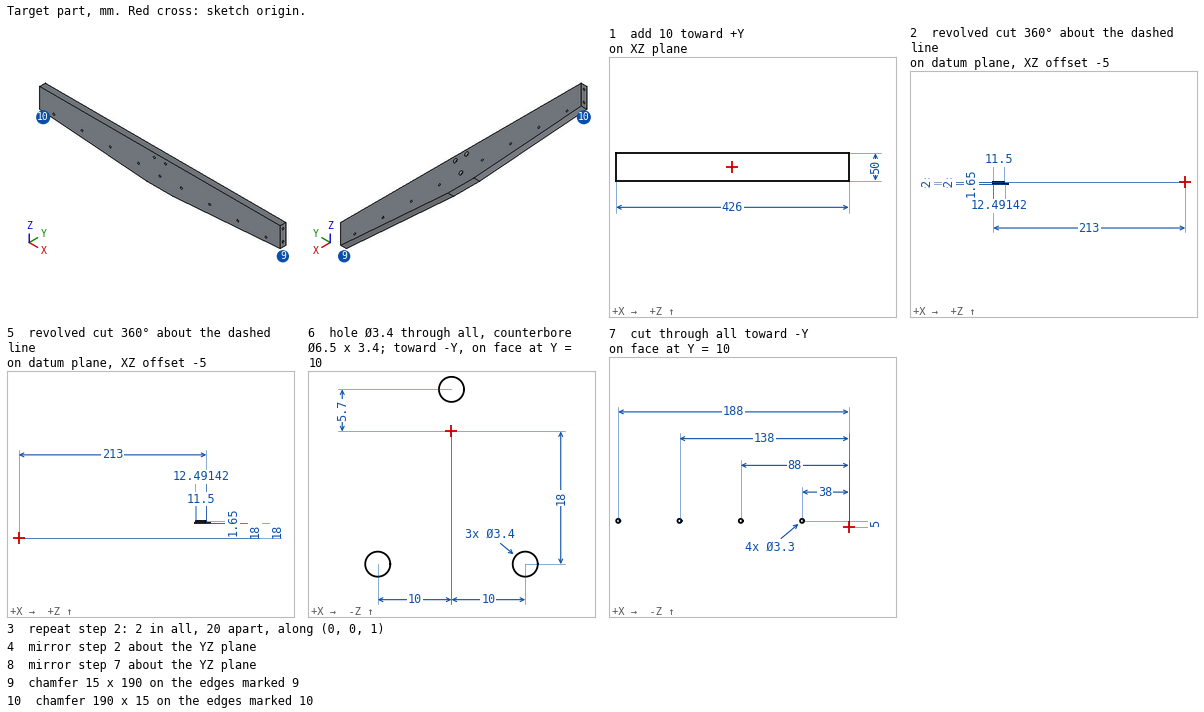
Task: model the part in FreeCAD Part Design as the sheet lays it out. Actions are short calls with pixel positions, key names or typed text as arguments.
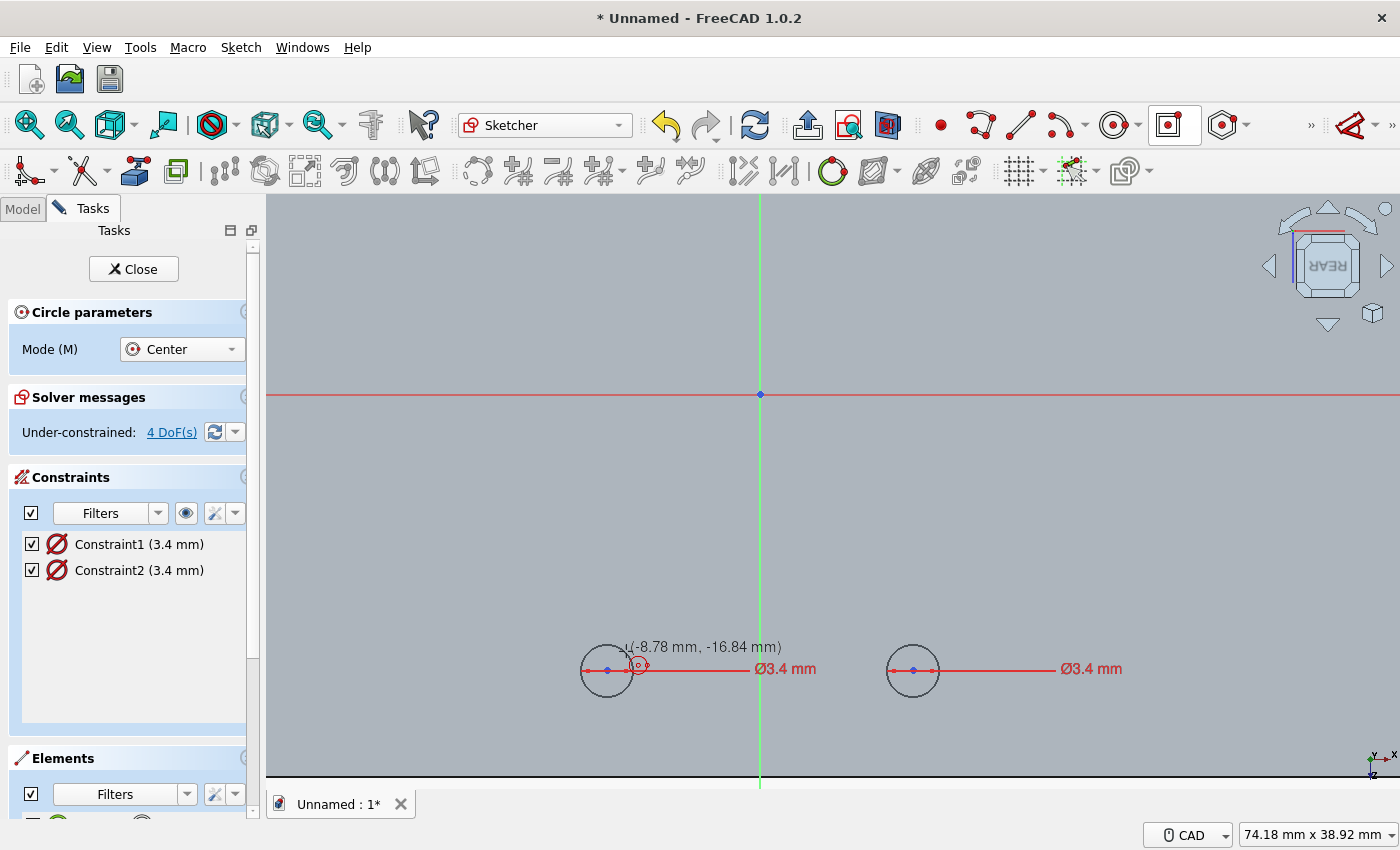
click(760, 307)
move(779, 289)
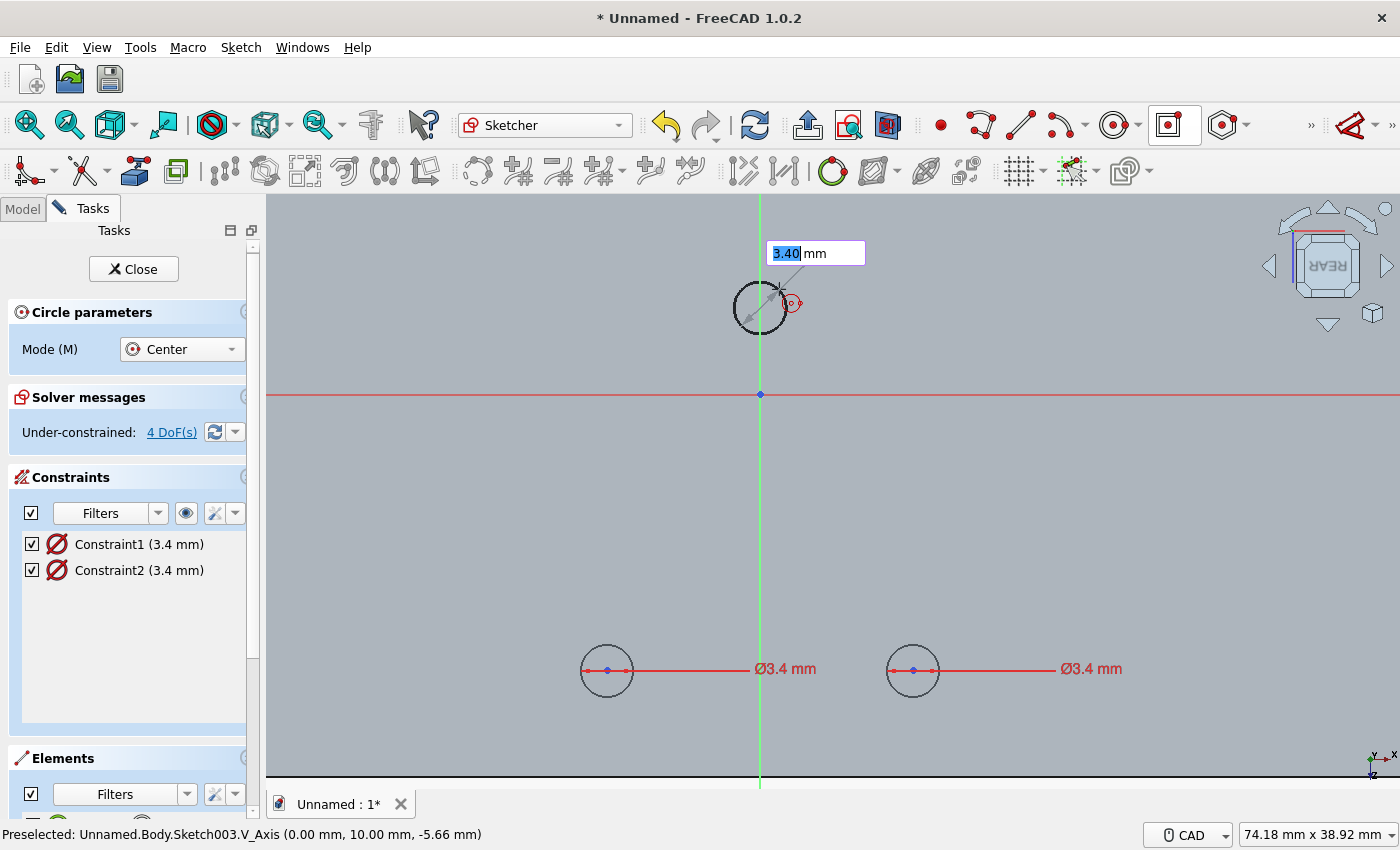
text(3.4)
key(Return)
key(Escape)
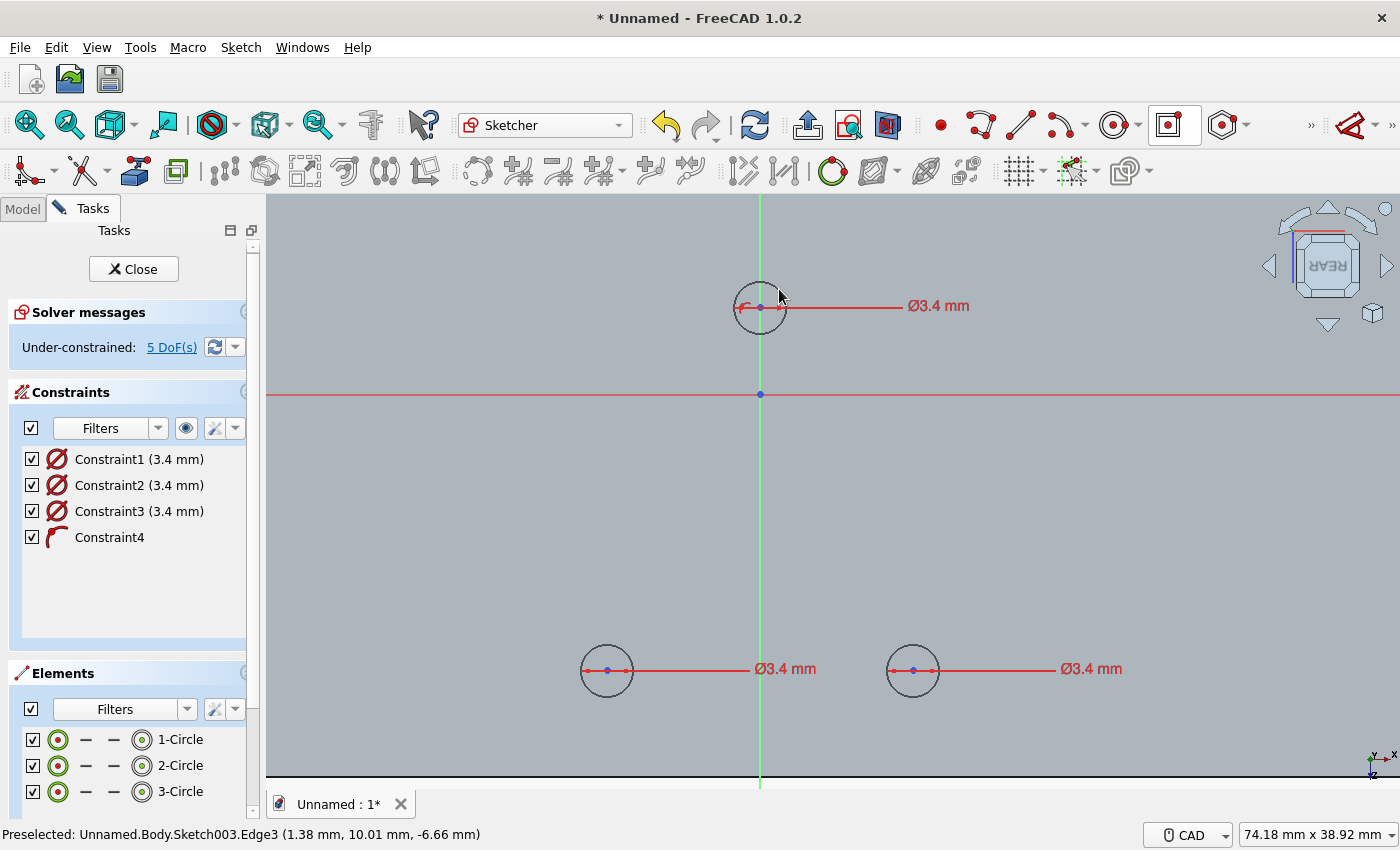
click(913, 671)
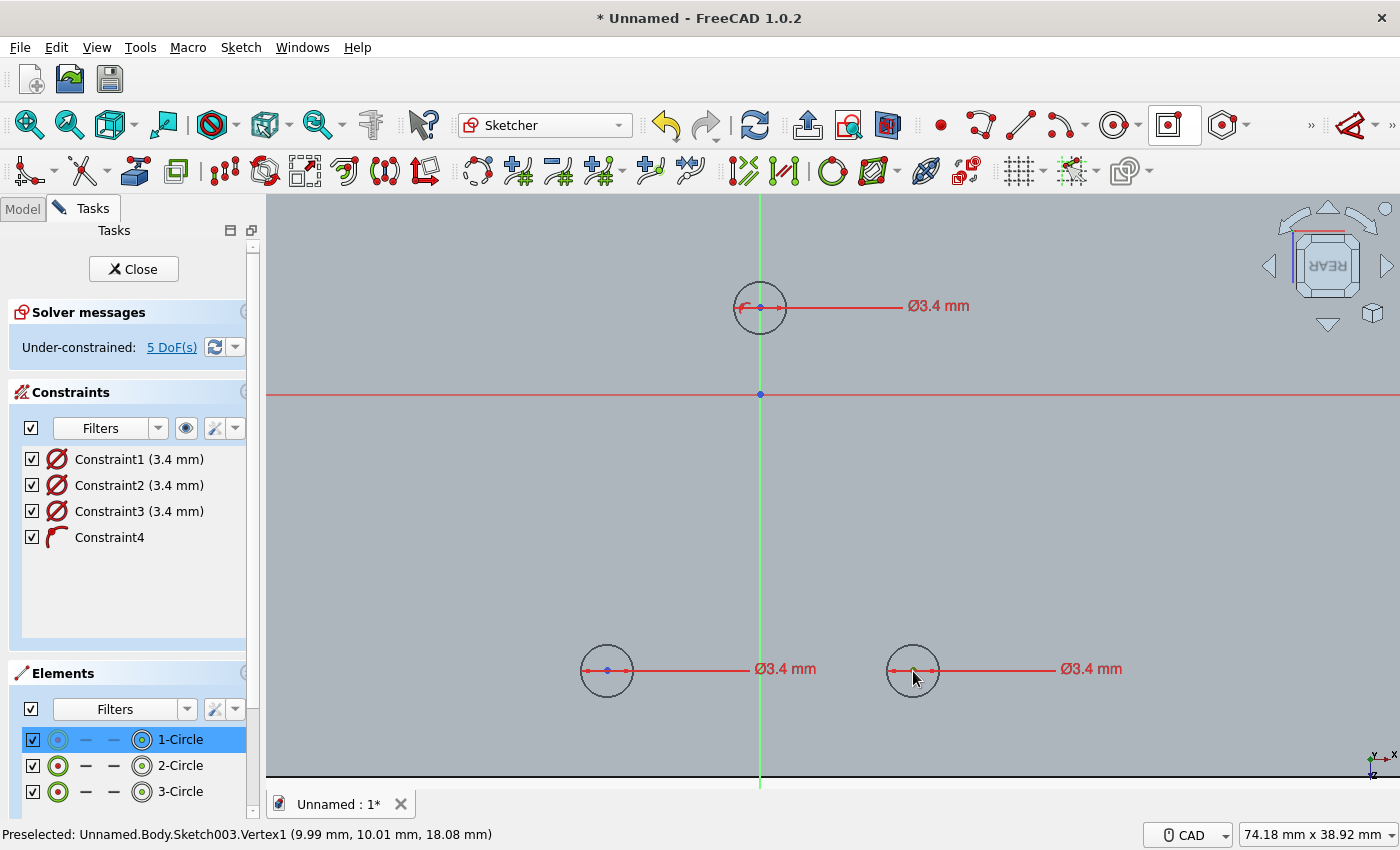
click(607, 671)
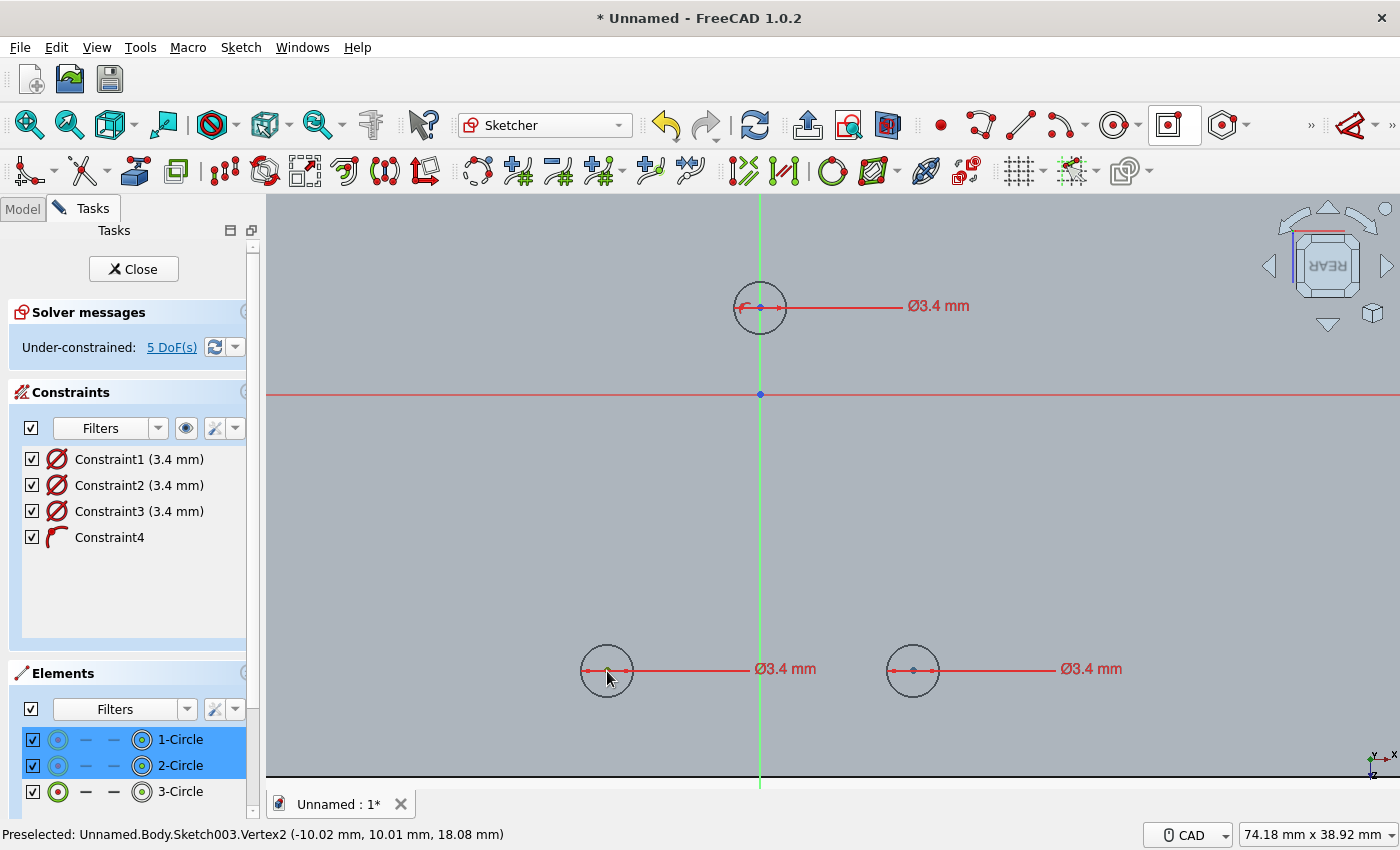
key(h)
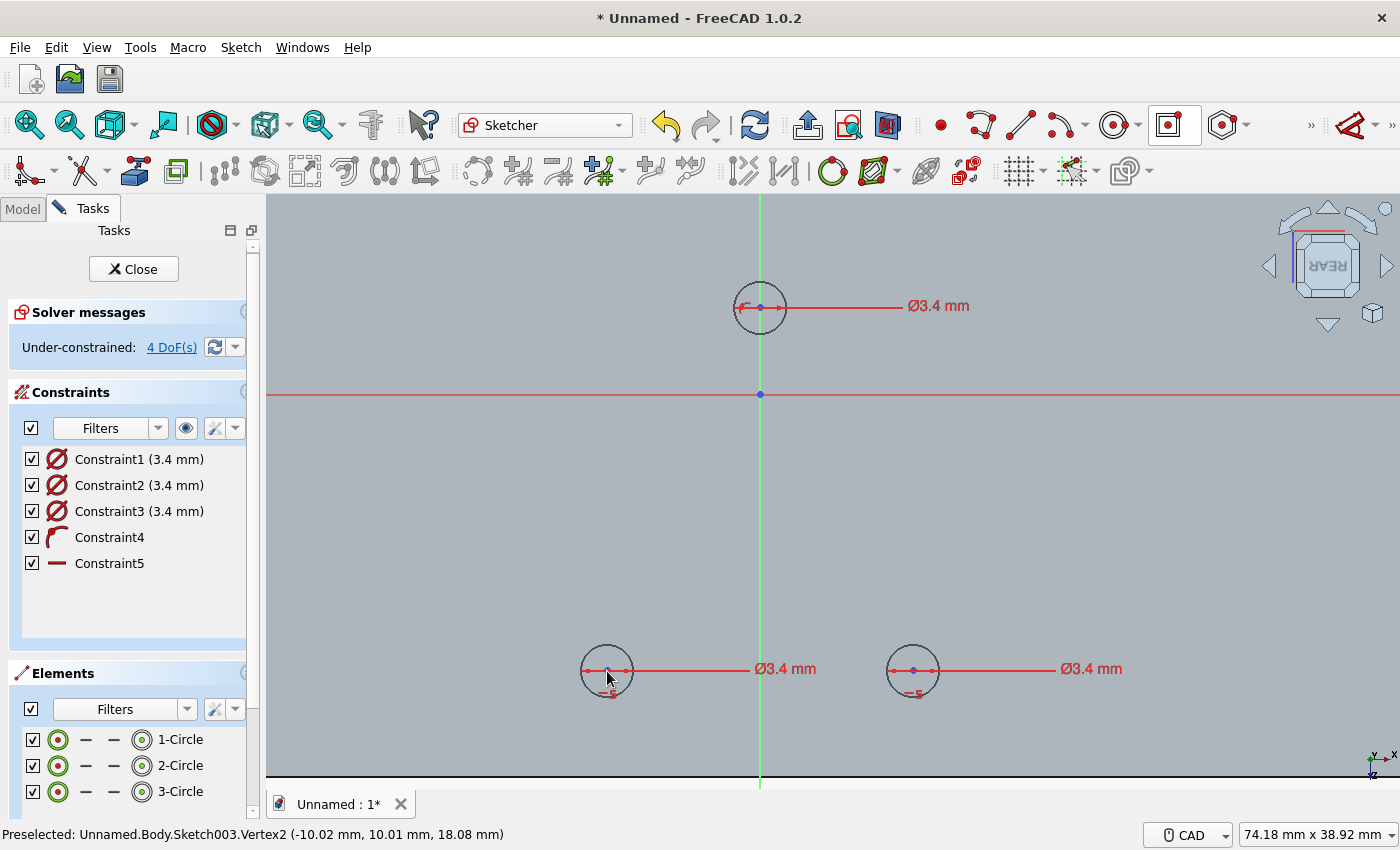
click(1350, 126)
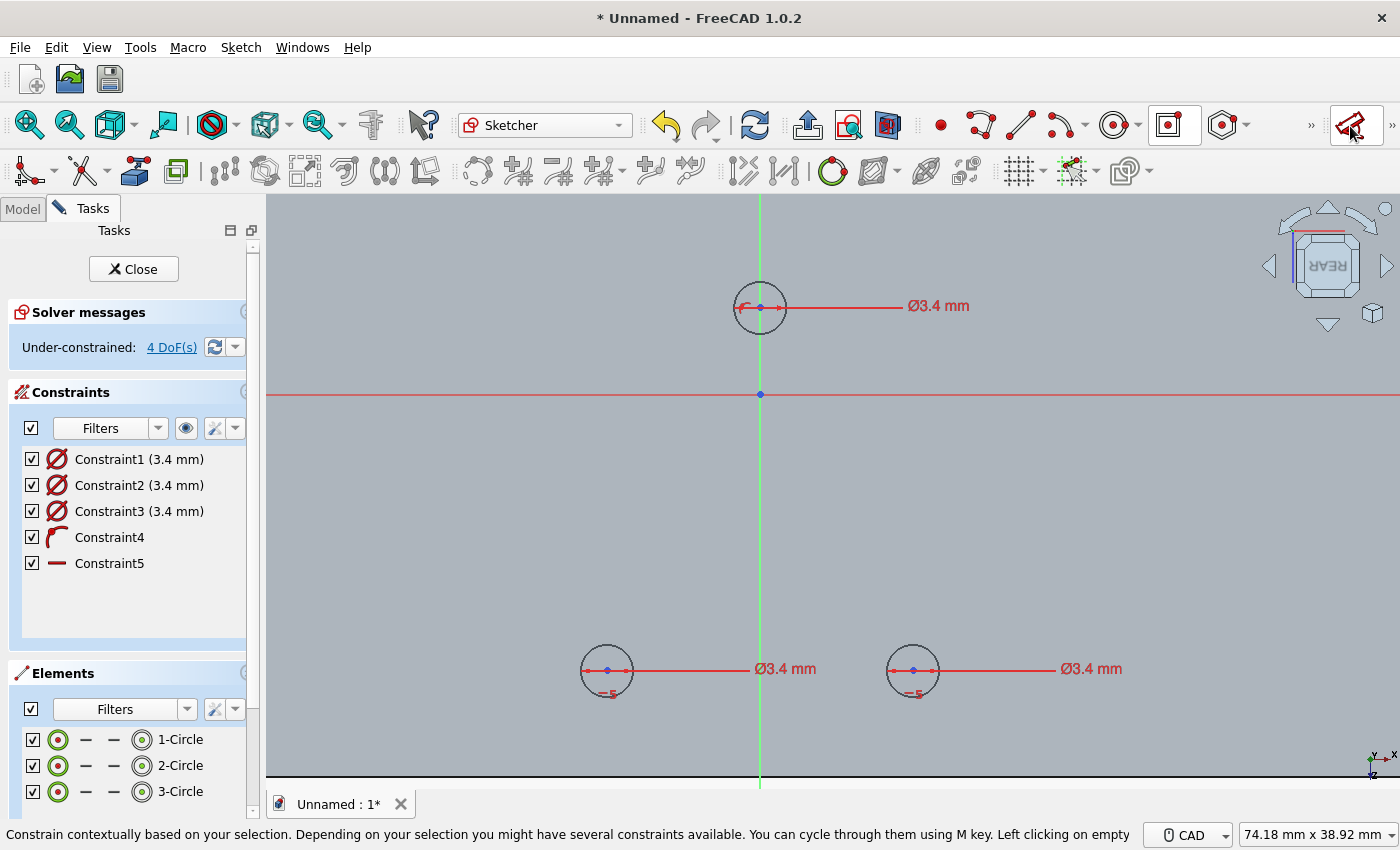
click(913, 671)
click(837, 705)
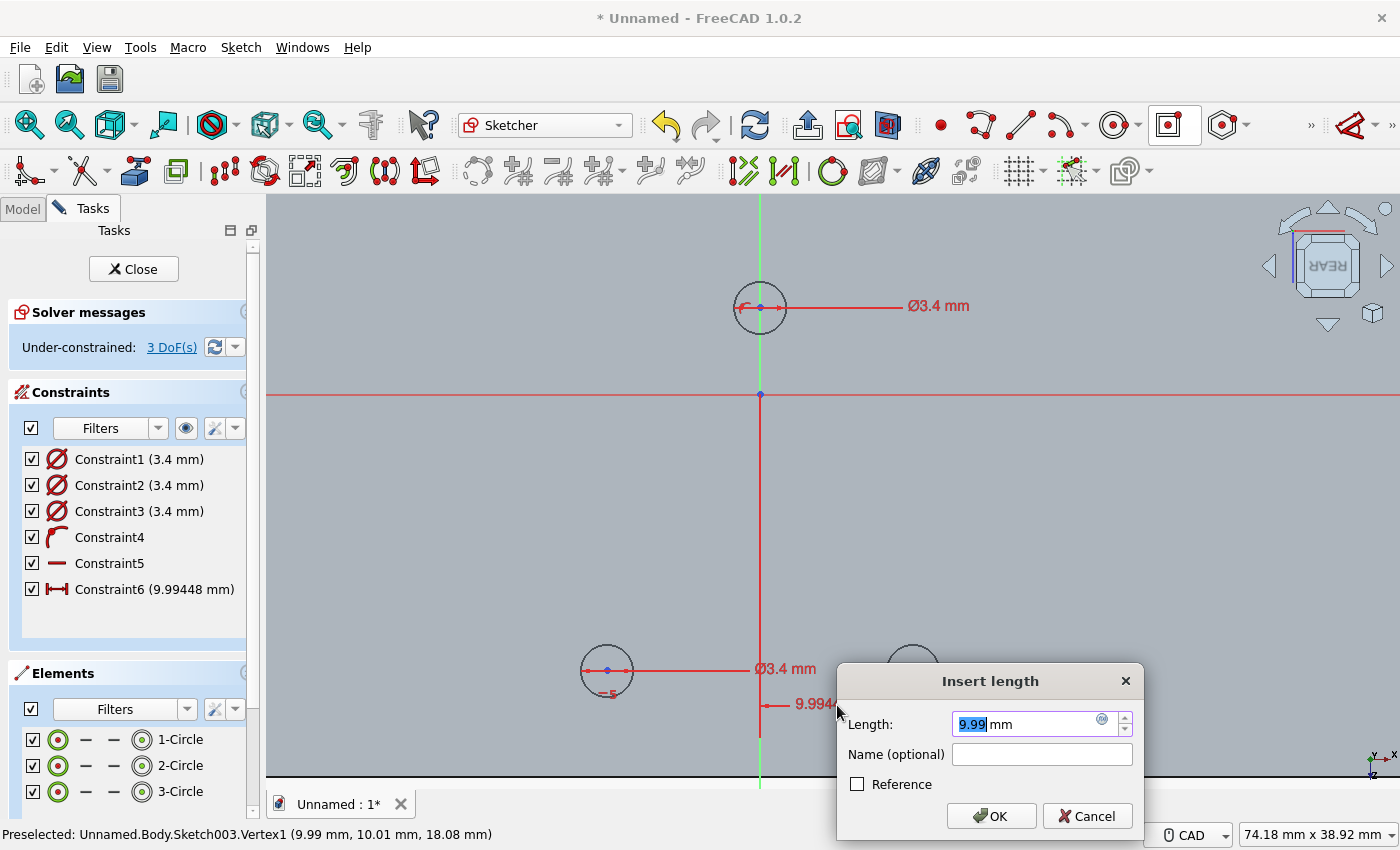
text(10)
key(Return)